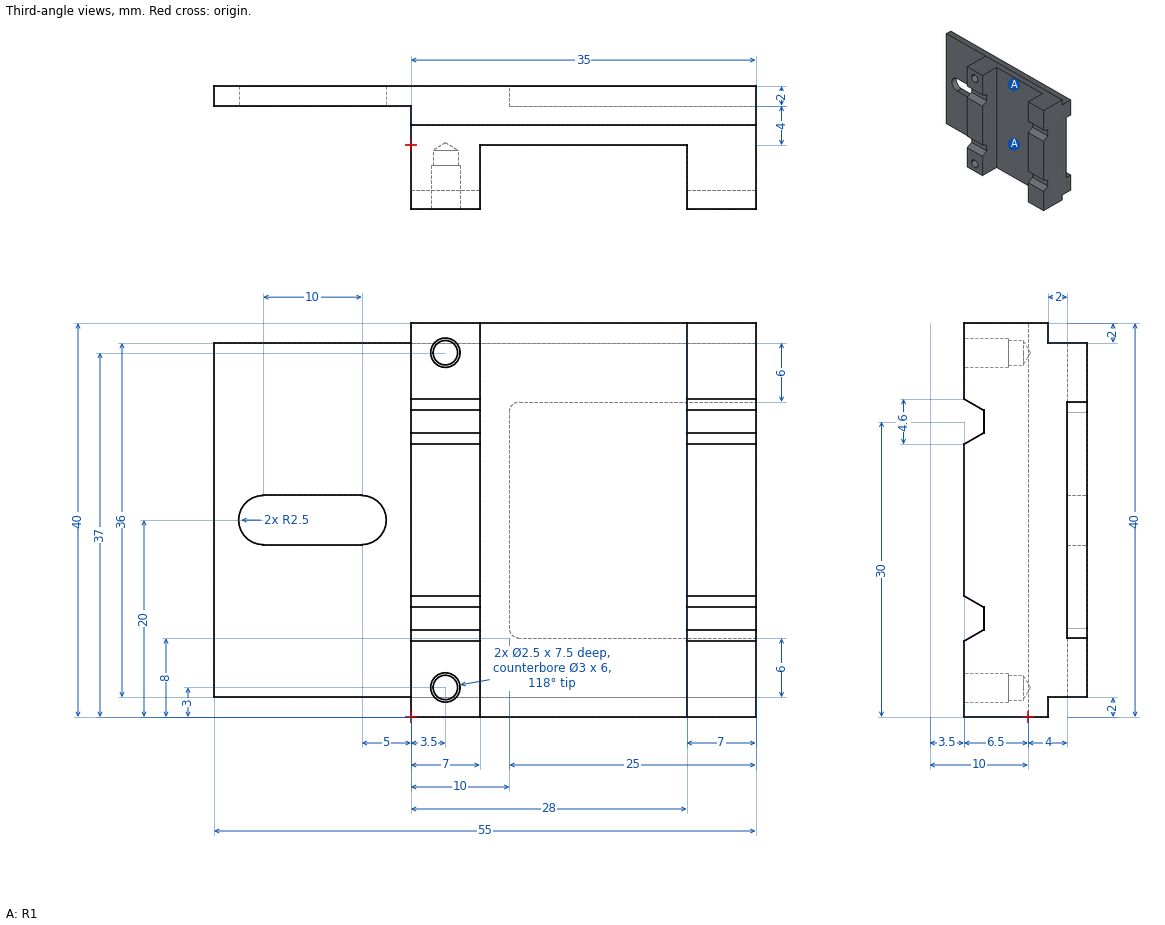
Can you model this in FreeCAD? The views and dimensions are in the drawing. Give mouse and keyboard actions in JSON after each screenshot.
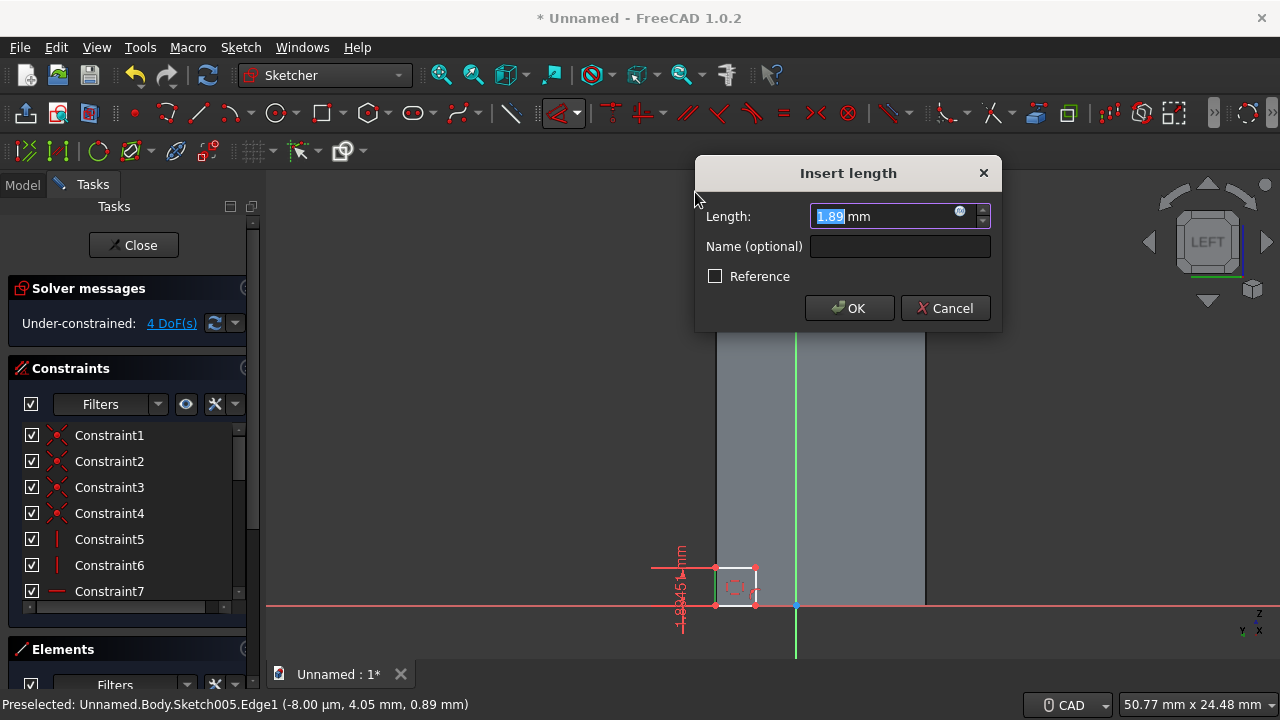
{"action": "type", "text": "2"}
{"action": "key", "text": "Return"}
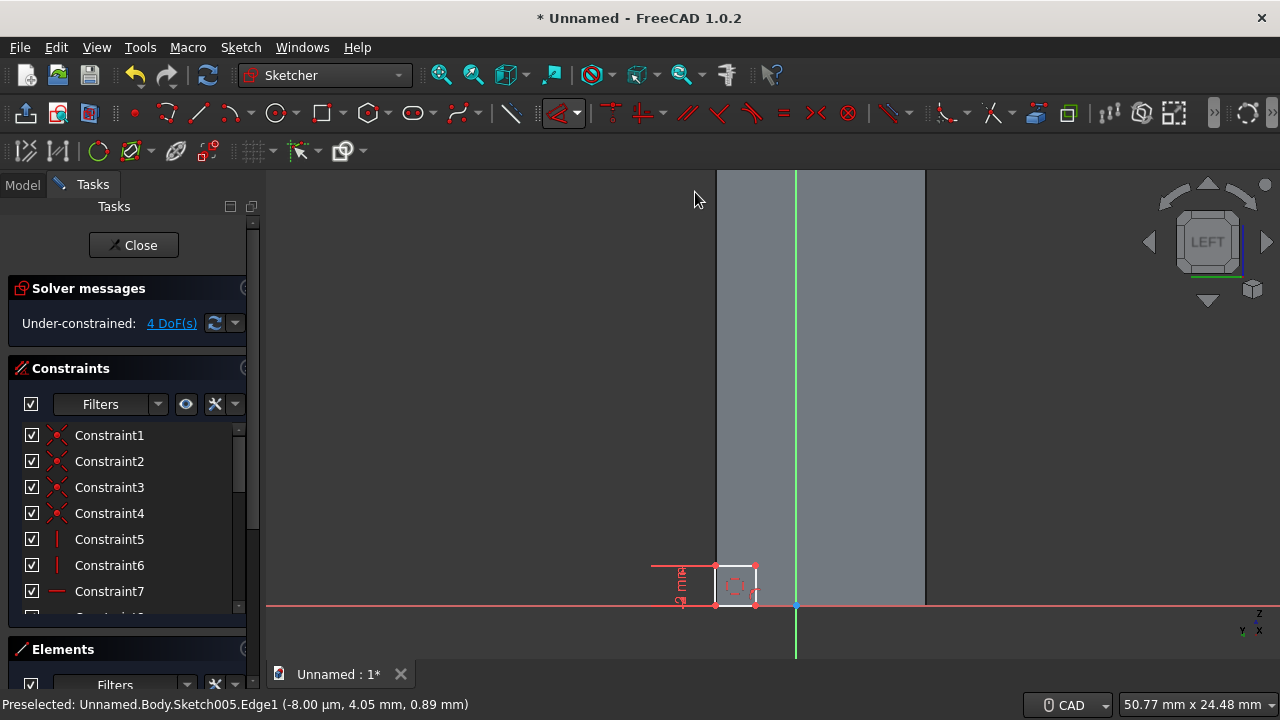
{"action": "left_click", "coordinate": [727, 606]}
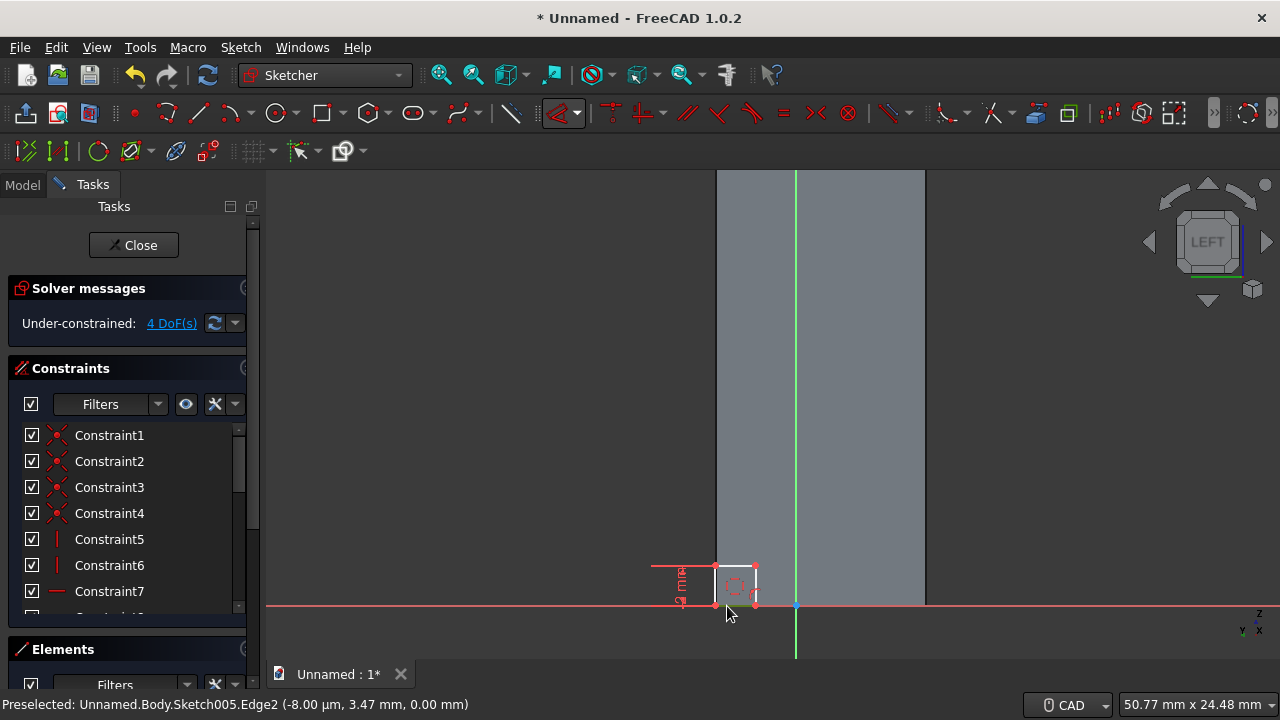
{"action": "left_click", "coordinate": [580, 114]}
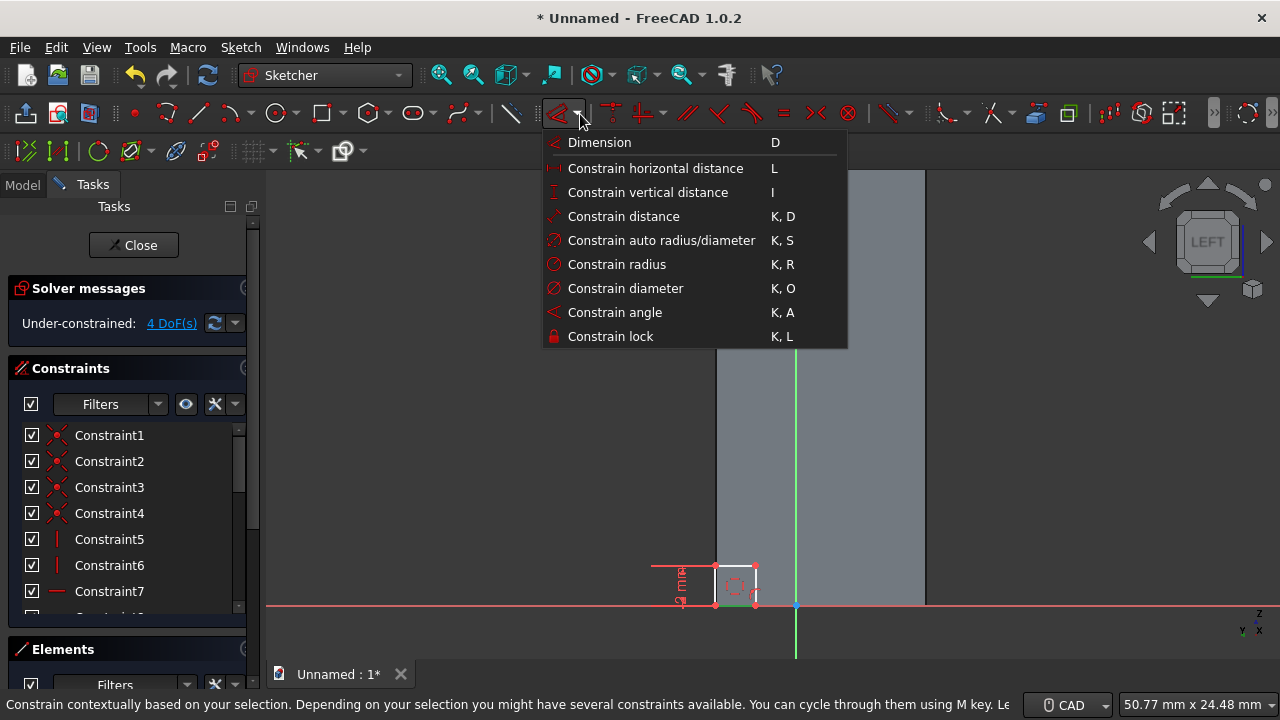
{"action": "left_click", "coordinate": [695, 168]}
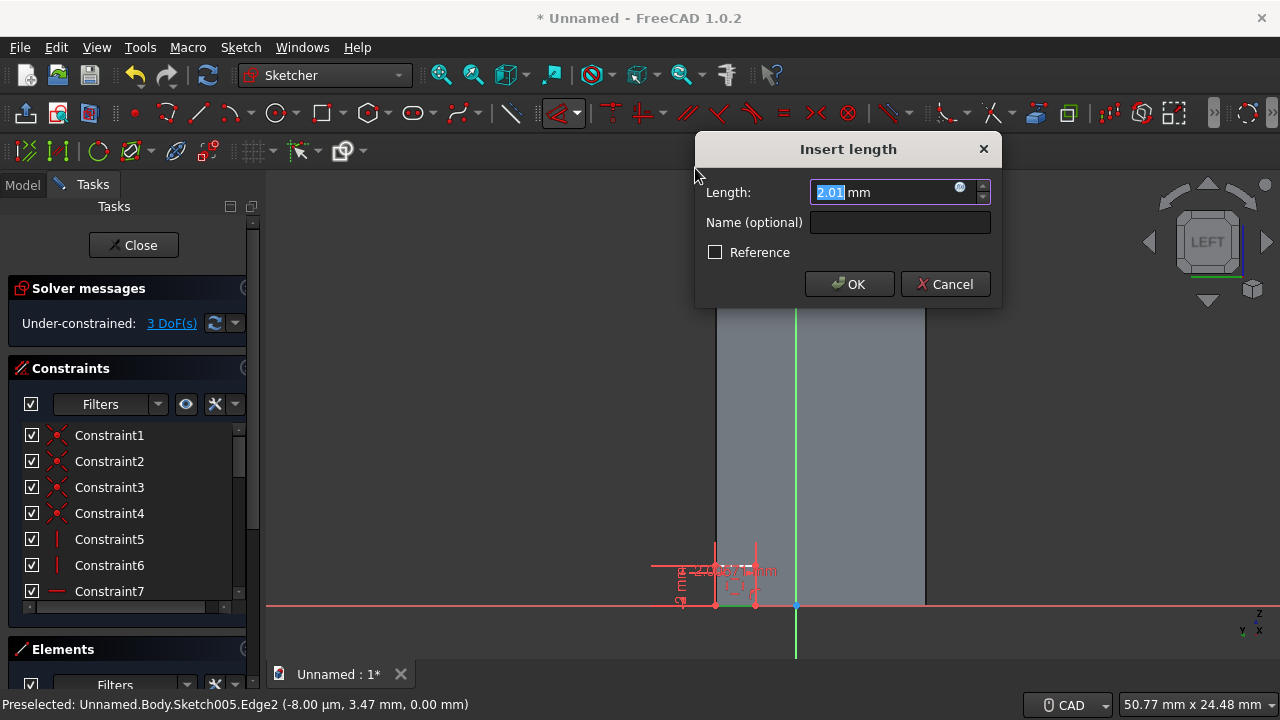
{"action": "type", "text": "2"}
{"action": "key", "text": "Return"}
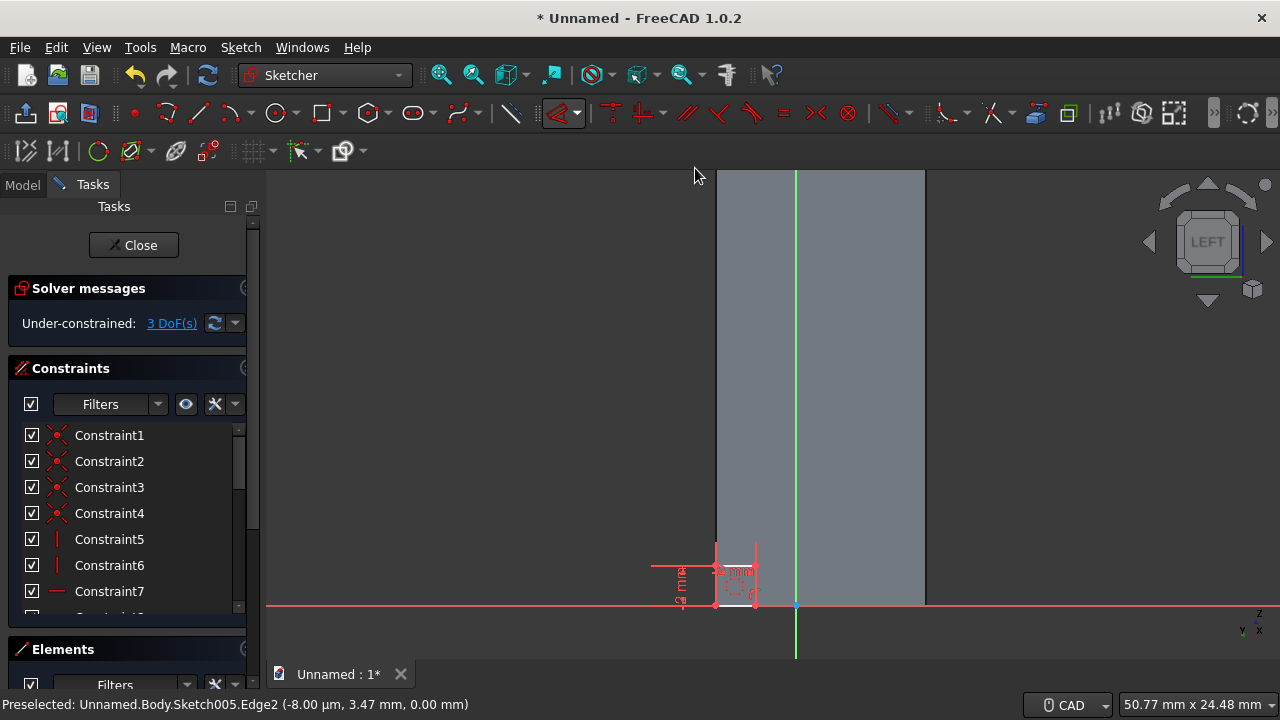
{"action": "left_click", "coordinate": [716, 566]}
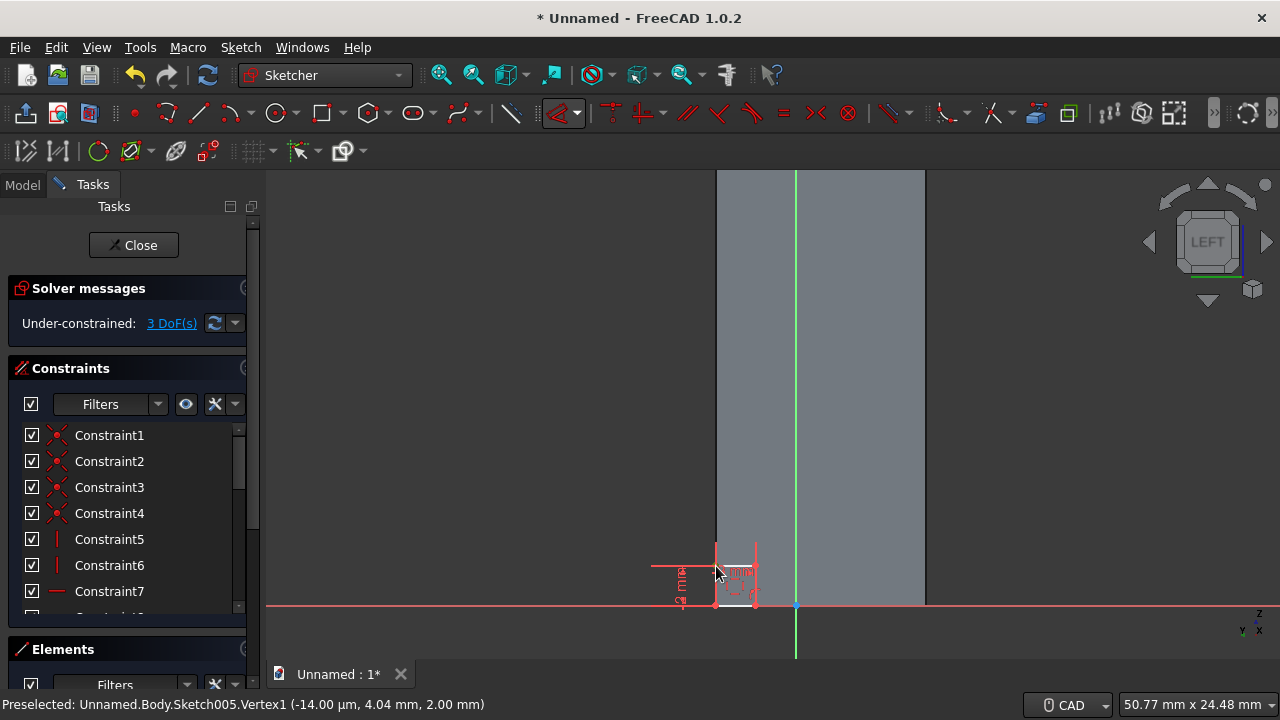
{"action": "left_click", "coordinate": [580, 114]}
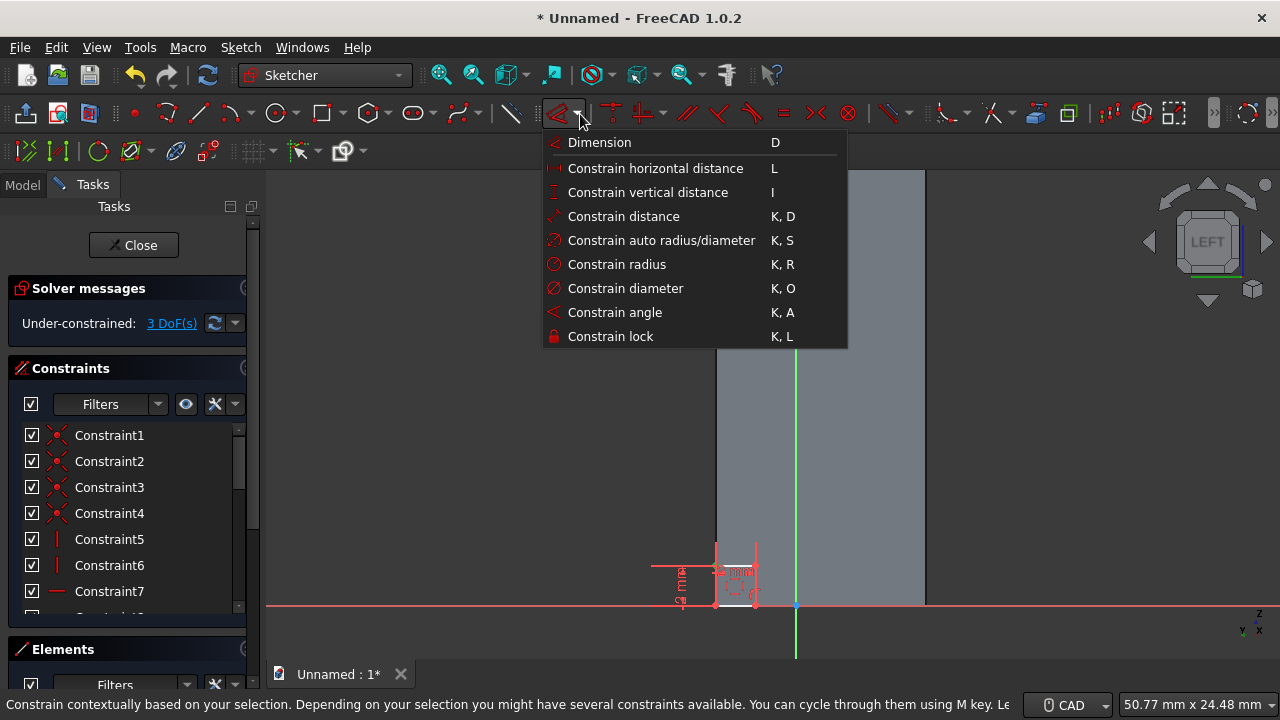
{"action": "left_click", "coordinate": [695, 168]}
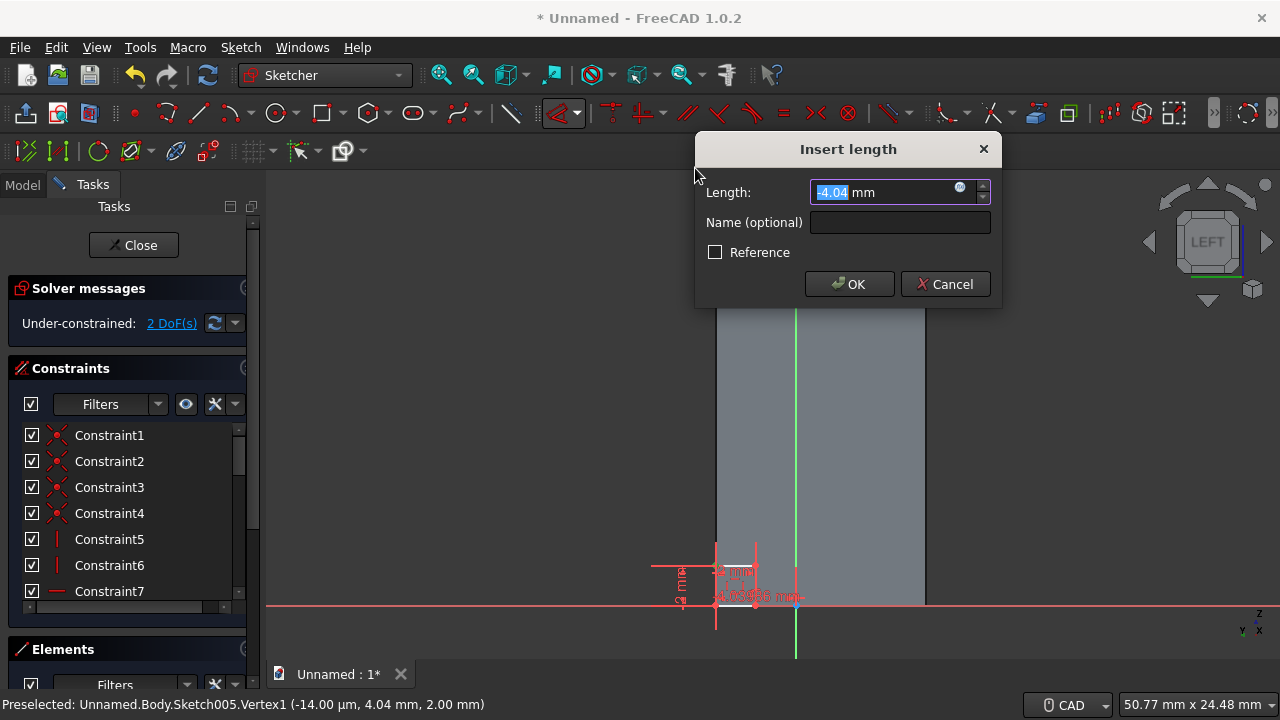
{"action": "type", "text": "-4"}
{"action": "key", "text": "Return"}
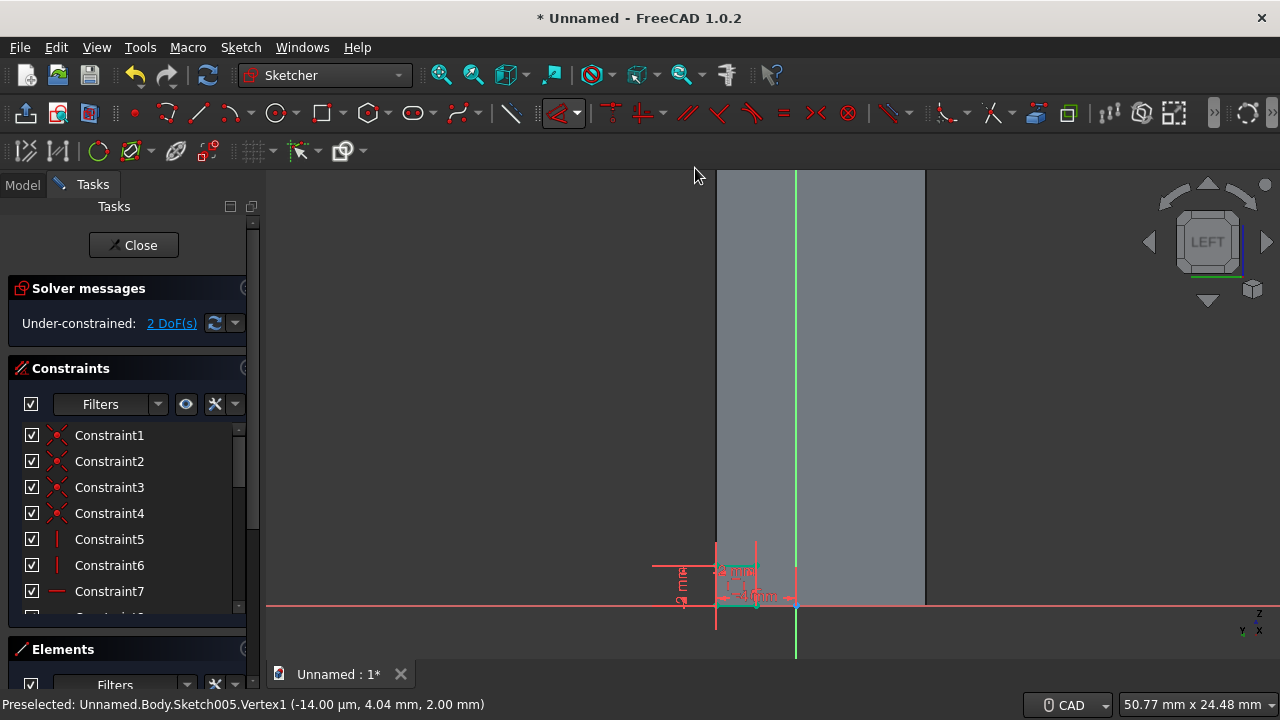
{"action": "scroll", "coordinate": [674, 536], "scroll_direction": "down", "scroll_amount": 5}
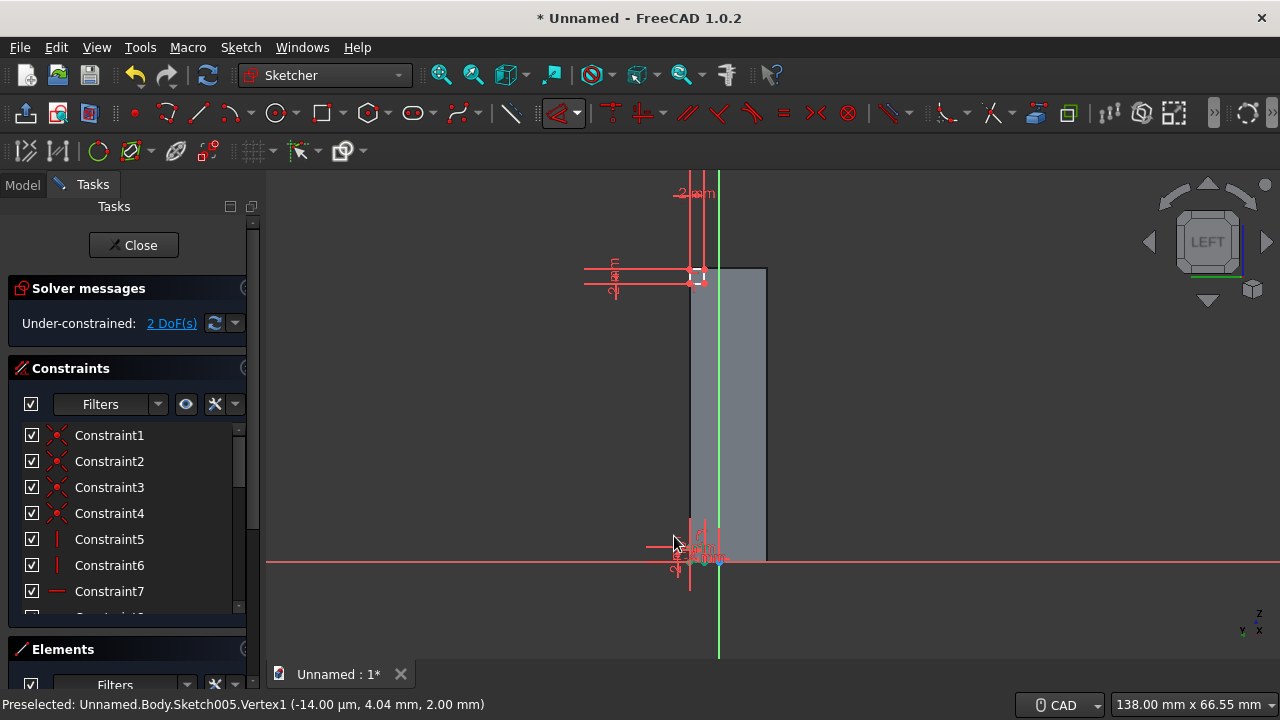
{"action": "scroll", "coordinate": [690, 269], "scroll_direction": "up", "scroll_amount": 2}